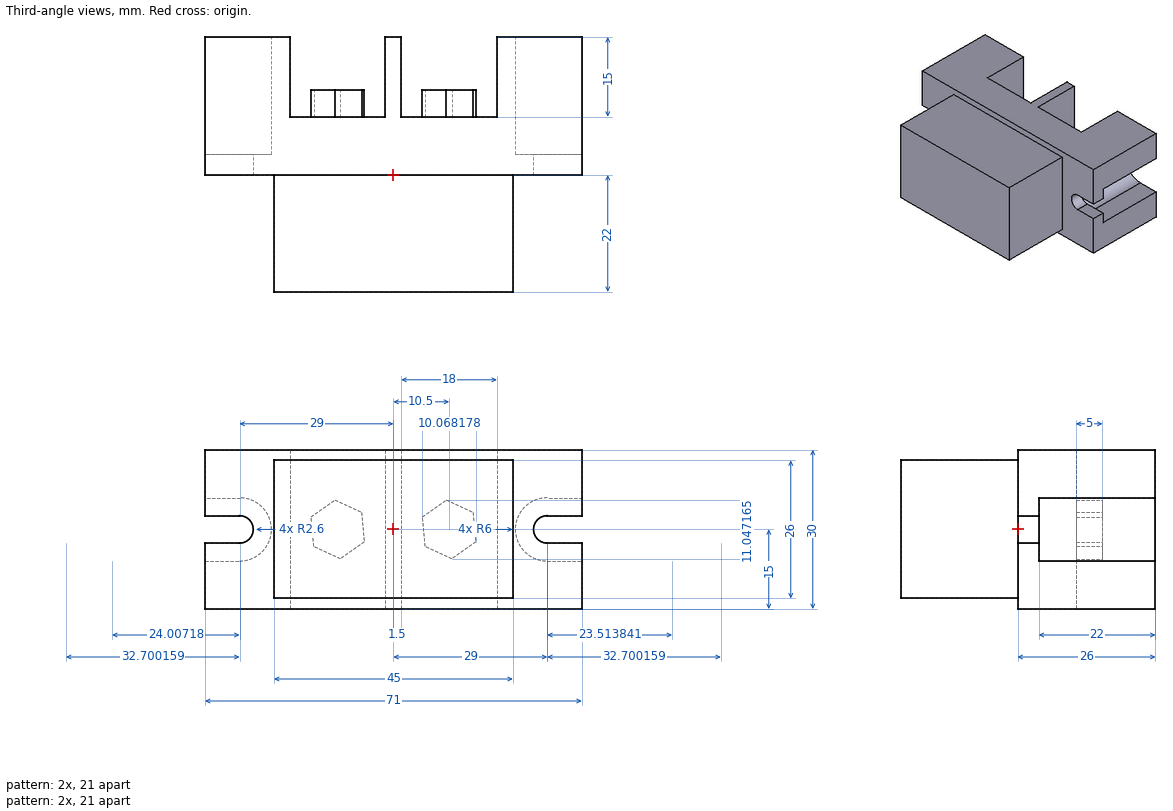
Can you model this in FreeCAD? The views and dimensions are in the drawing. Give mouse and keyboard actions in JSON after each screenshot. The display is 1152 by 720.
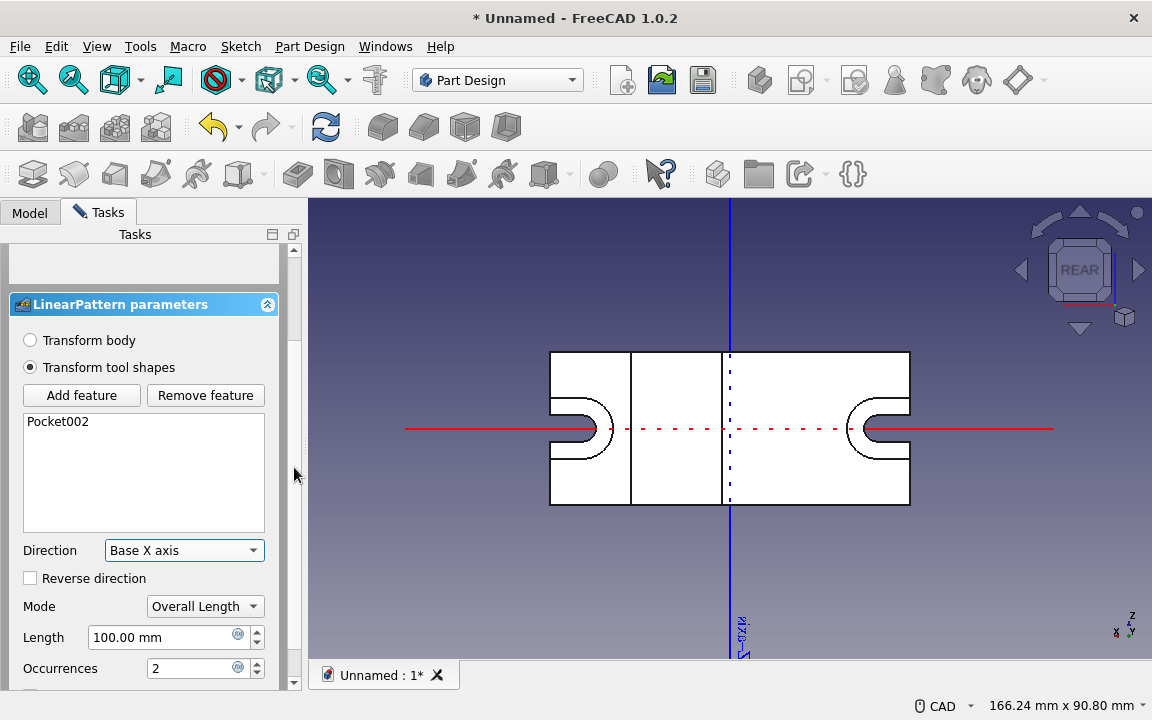
{"action": "left_click", "coordinate": [206, 606]}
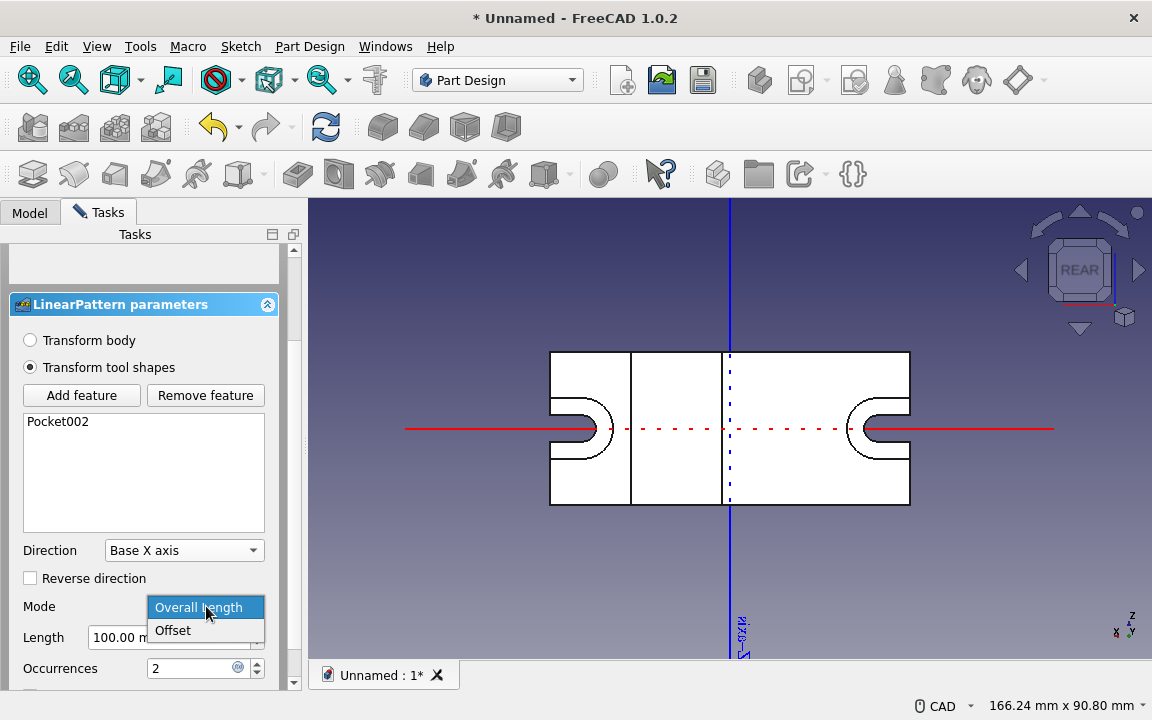
{"action": "left_click", "coordinate": [204, 630]}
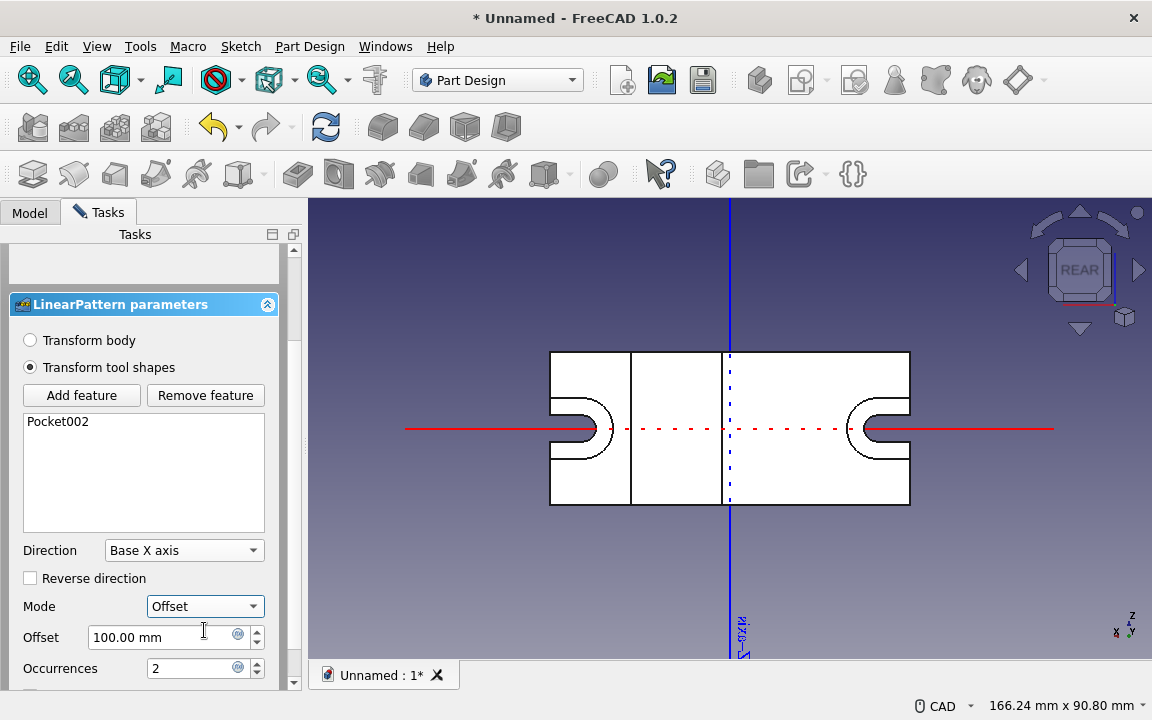
{"action": "triple_click", "coordinate": [170, 638]}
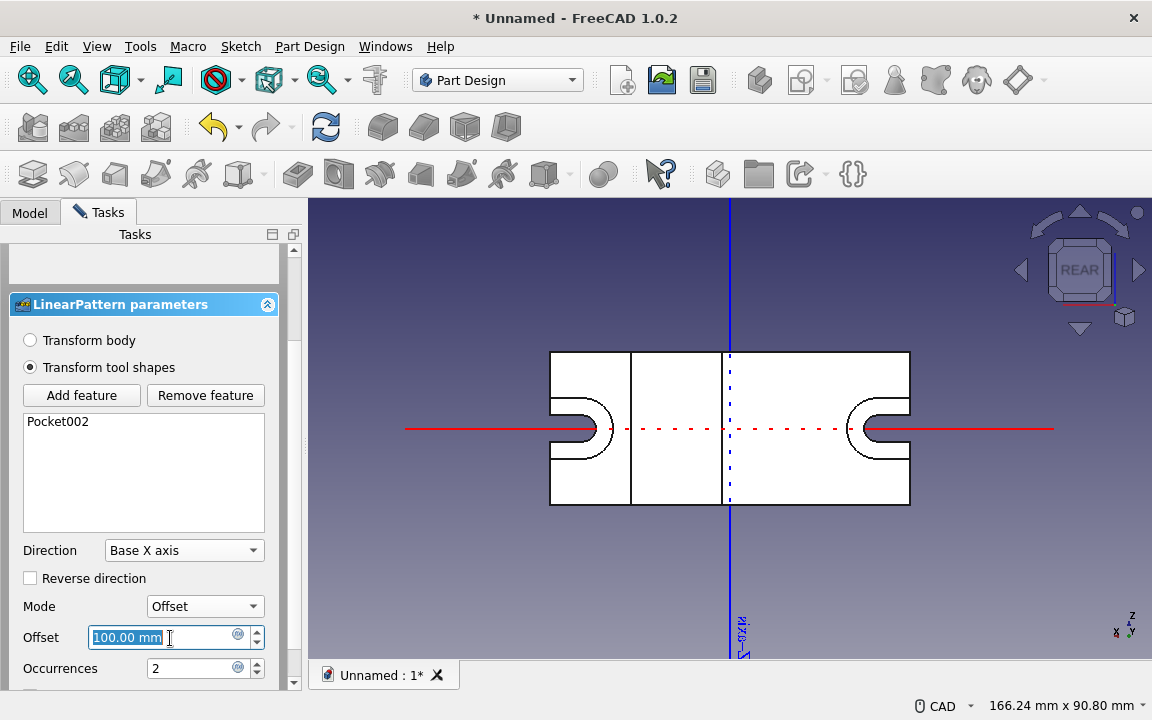
{"action": "type", "text": "21"}
{"action": "key", "text": "Tab"}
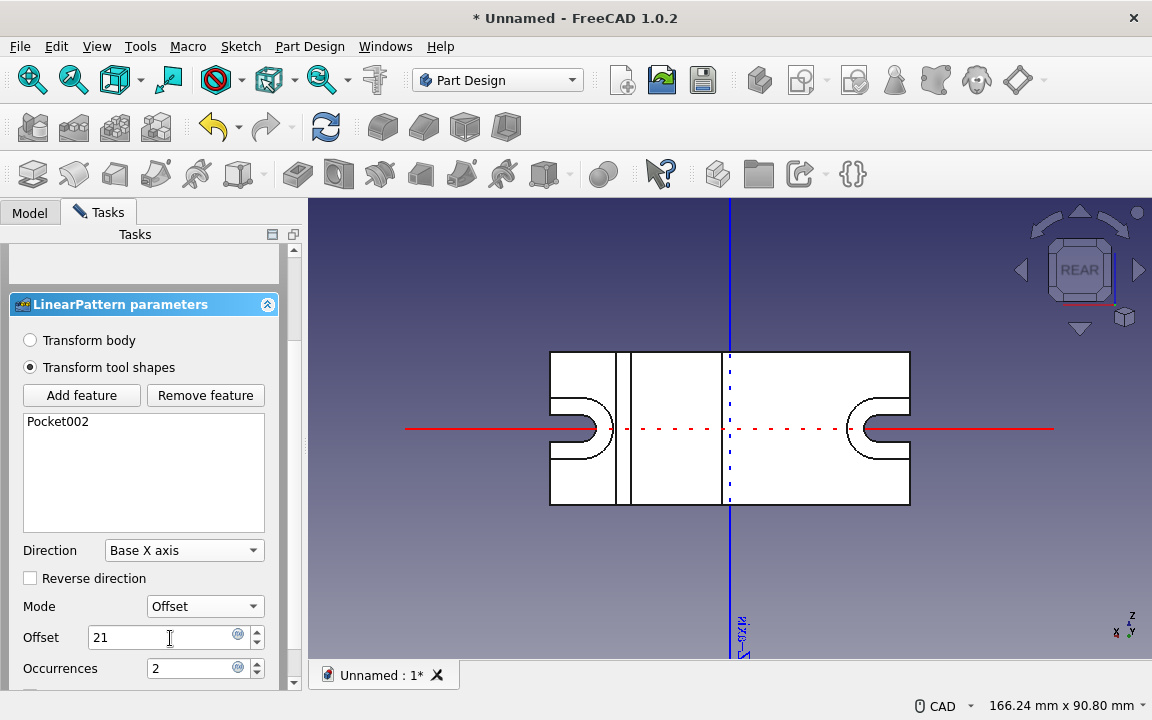
{"action": "triple_click", "coordinate": [199, 668]}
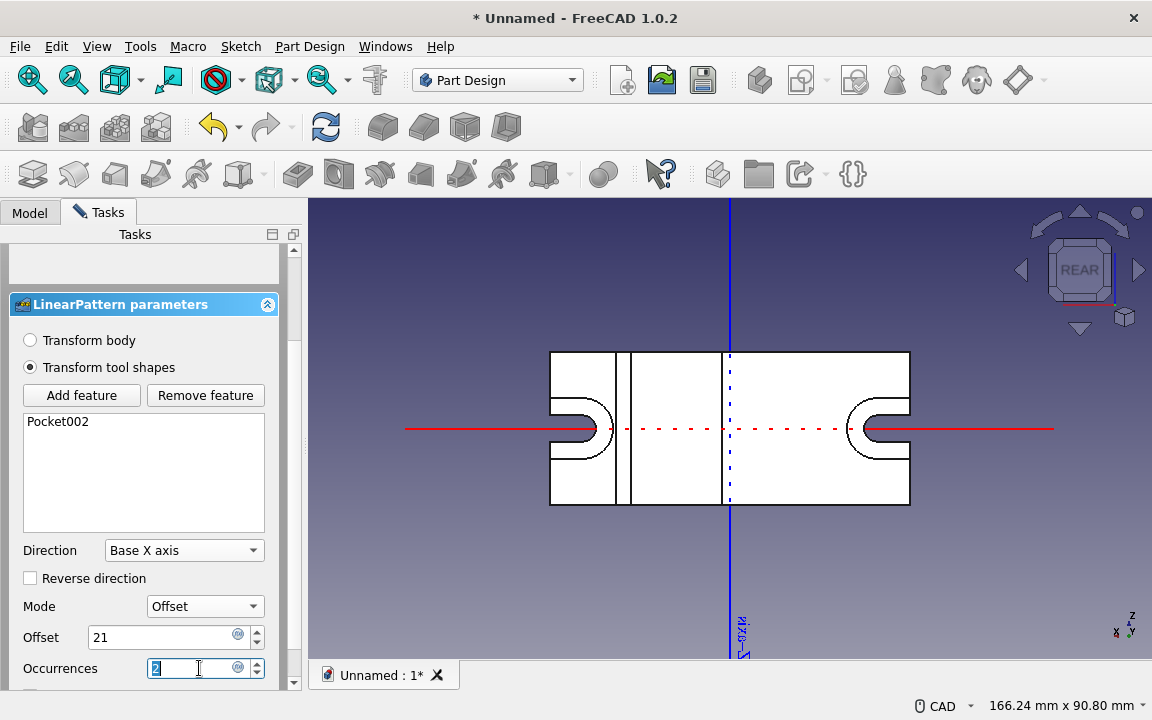
{"action": "type", "text": "2"}
{"action": "key", "text": "Tab"}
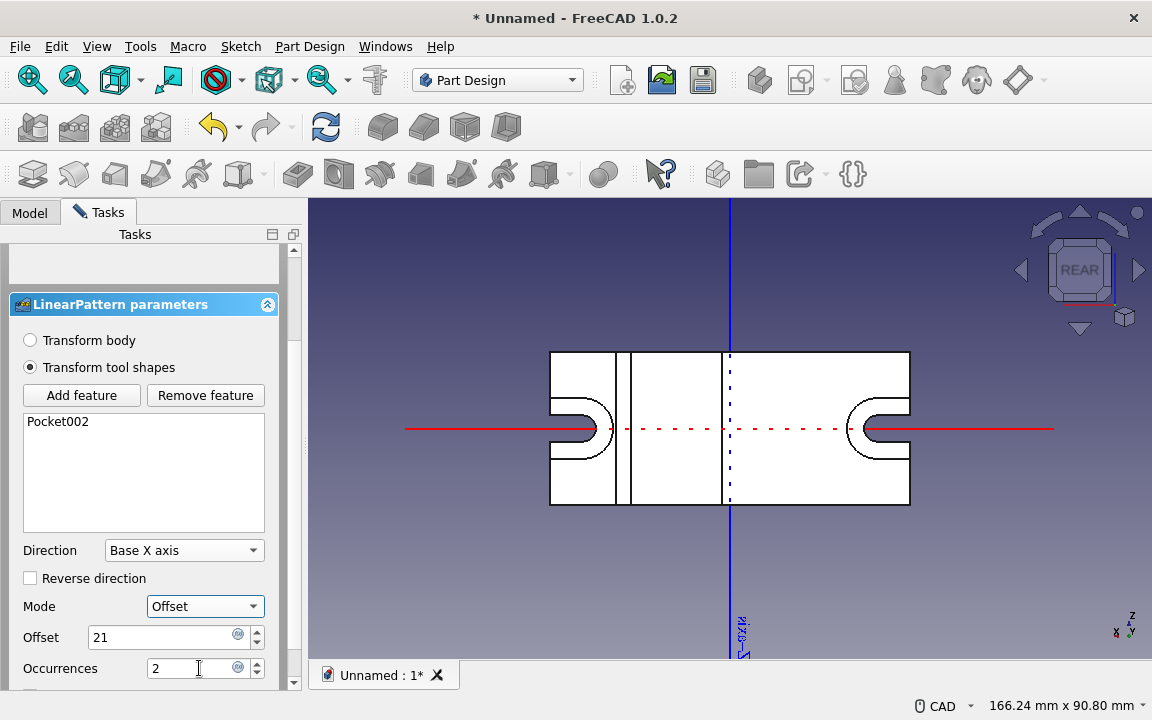
{"action": "left_click", "coordinate": [31, 578]}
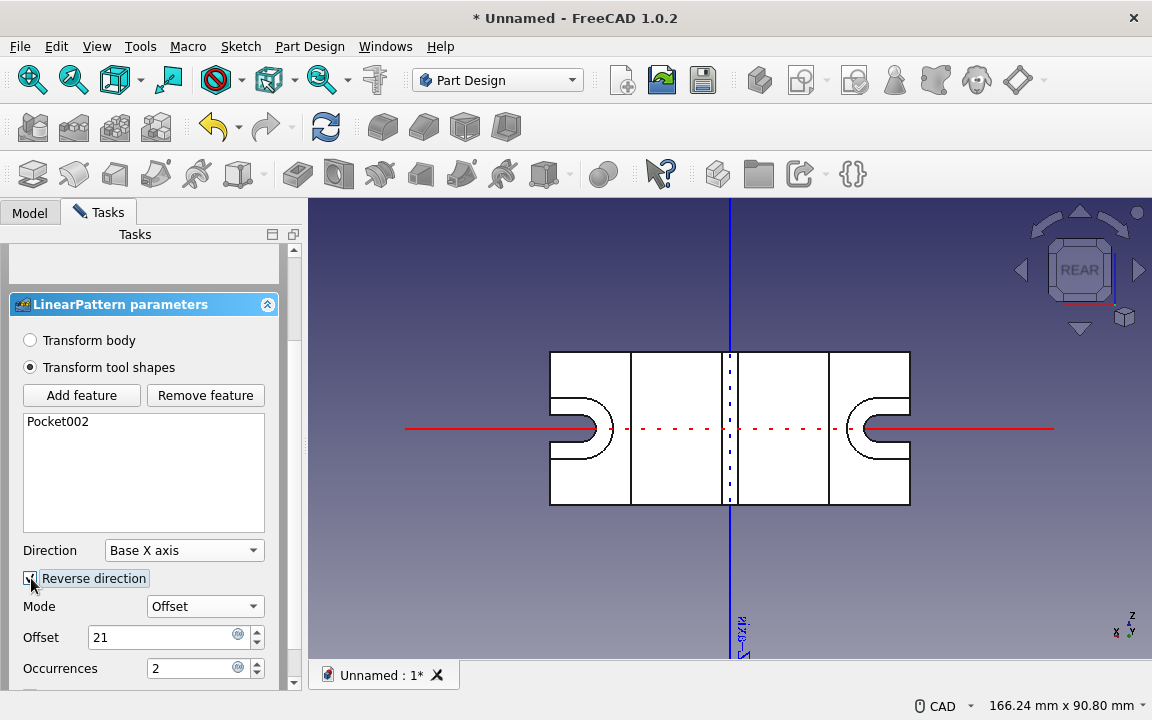
{"action": "scroll", "coordinate": [294, 467], "scroll_direction": "up", "scroll_amount": 3}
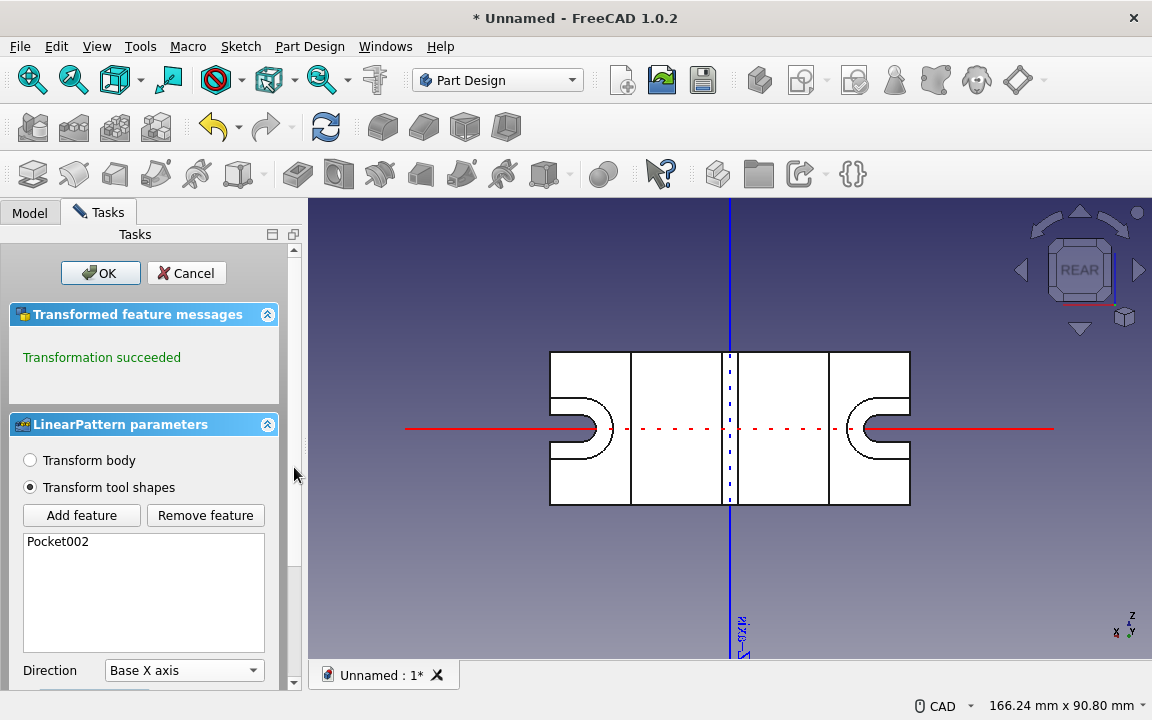
{"action": "left_click", "coordinate": [101, 273]}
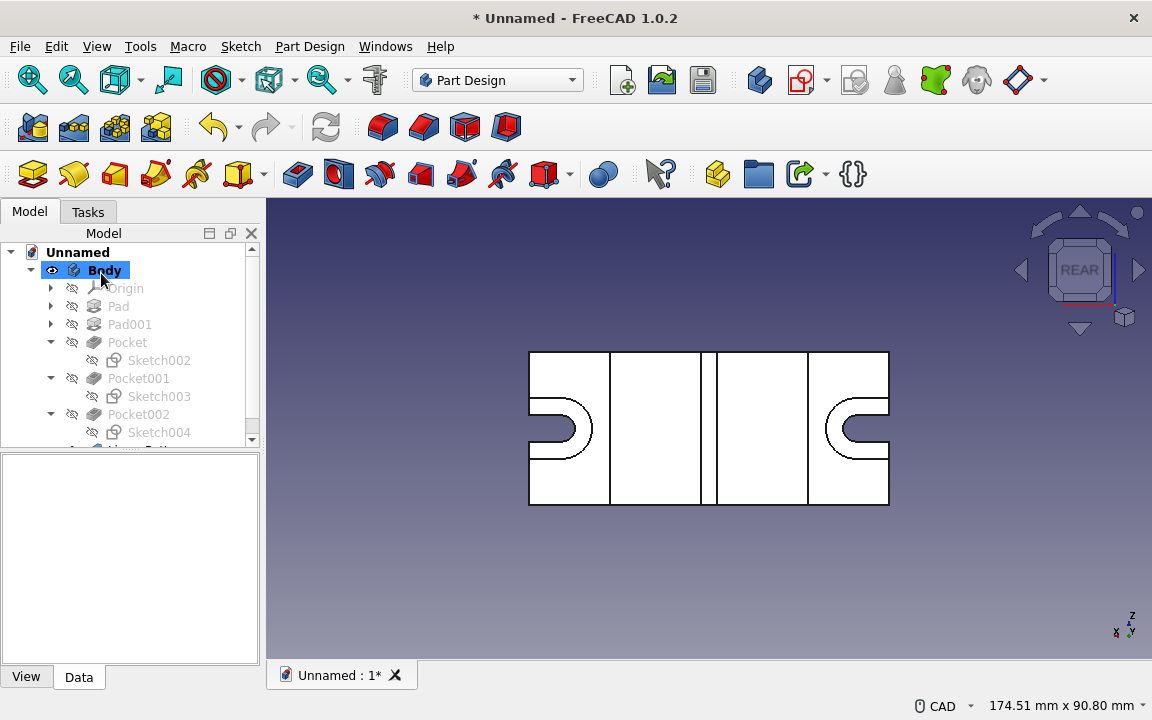
{"action": "left_click", "coordinate": [33, 80]}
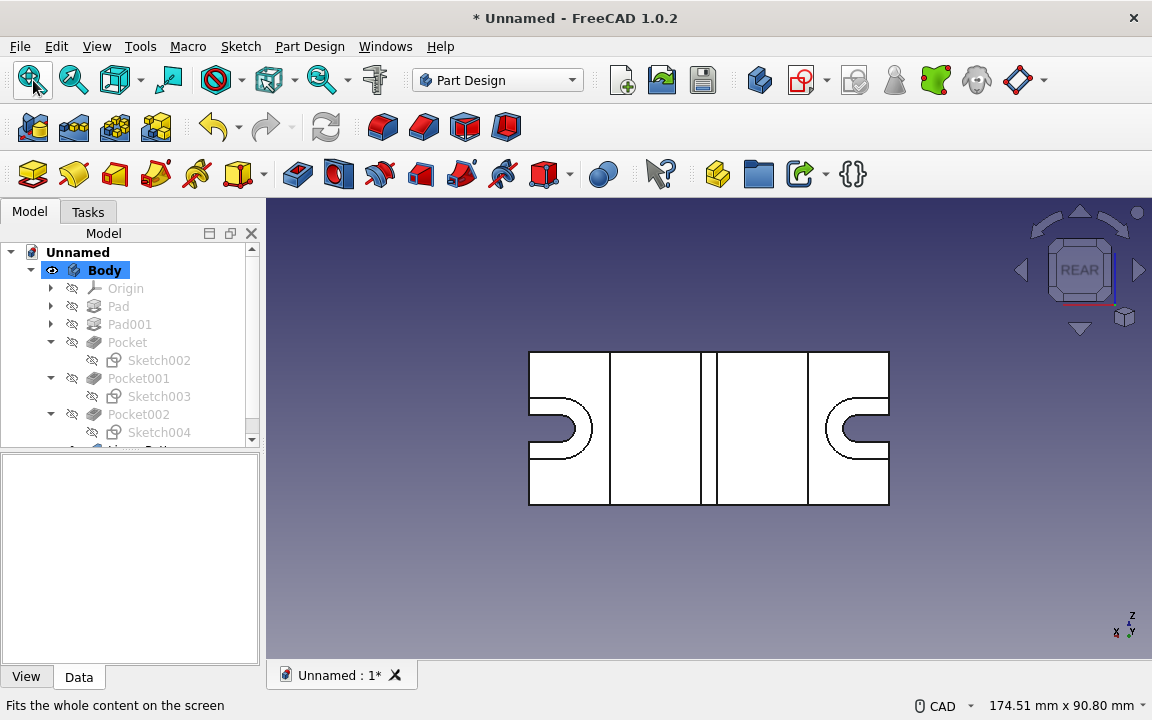
{"action": "left_click", "coordinate": [656, 406]}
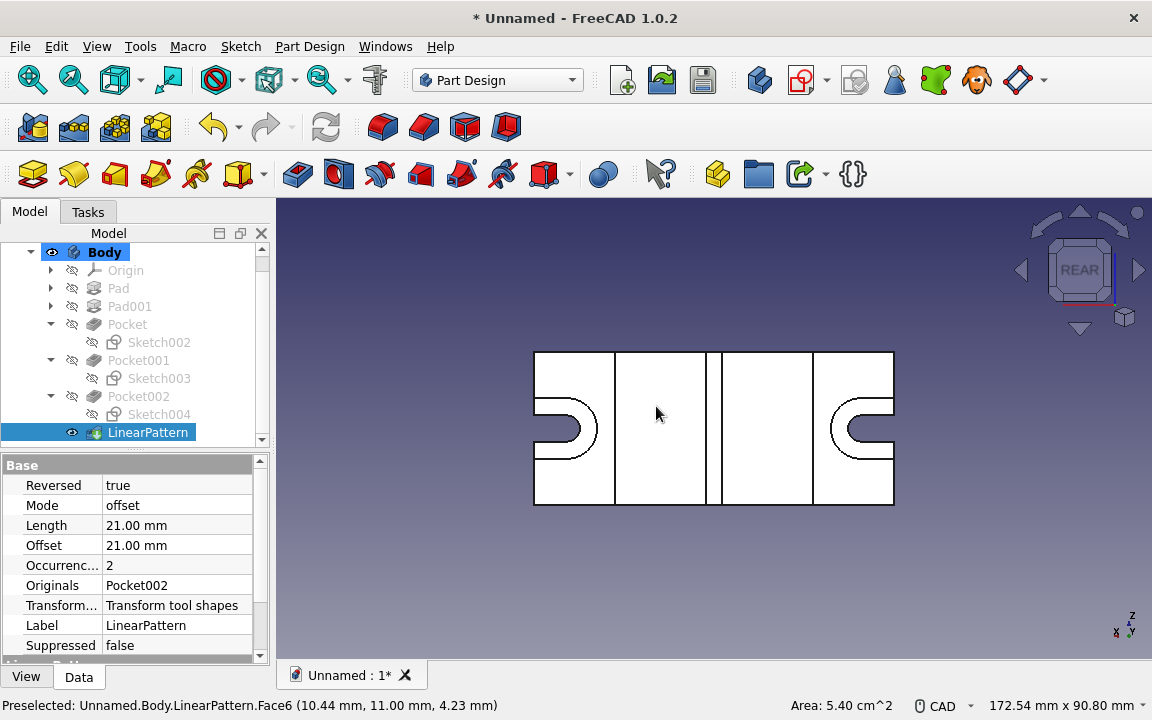
{"action": "left_click", "coordinate": [800, 80]}